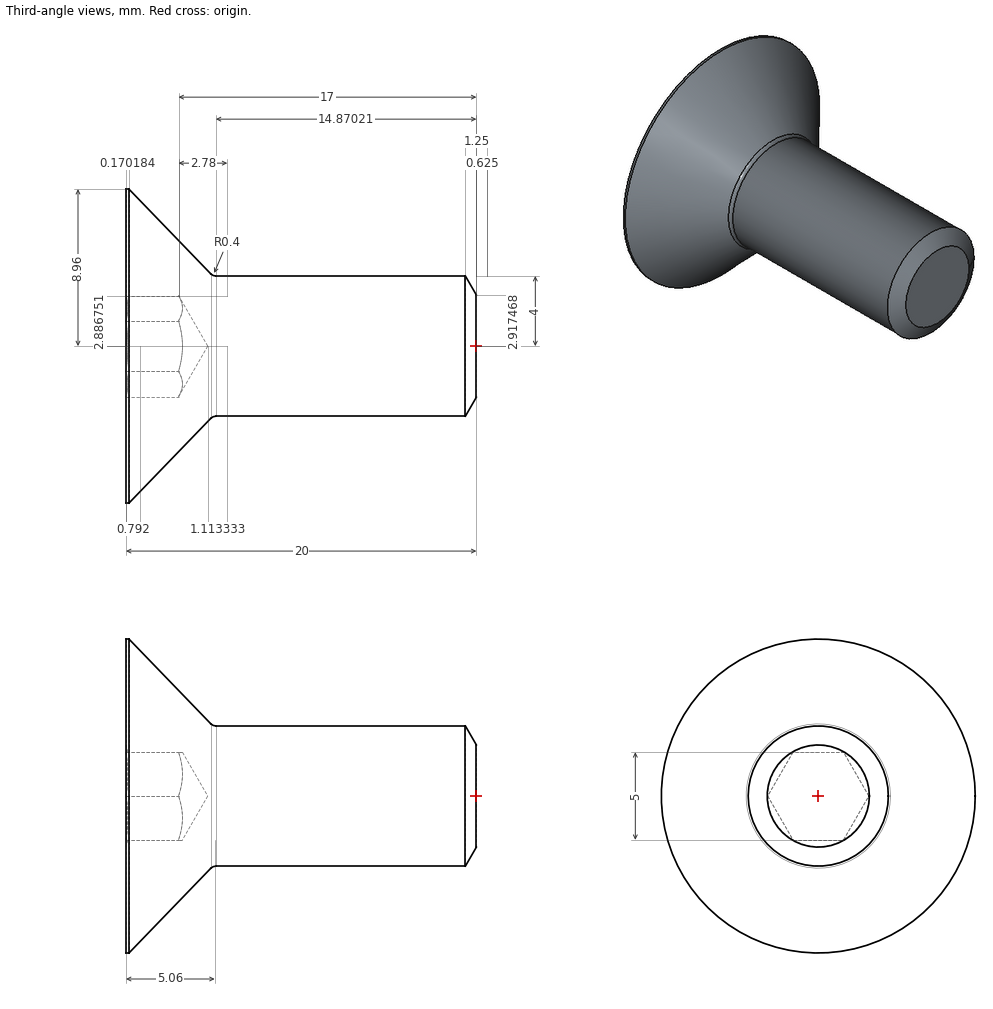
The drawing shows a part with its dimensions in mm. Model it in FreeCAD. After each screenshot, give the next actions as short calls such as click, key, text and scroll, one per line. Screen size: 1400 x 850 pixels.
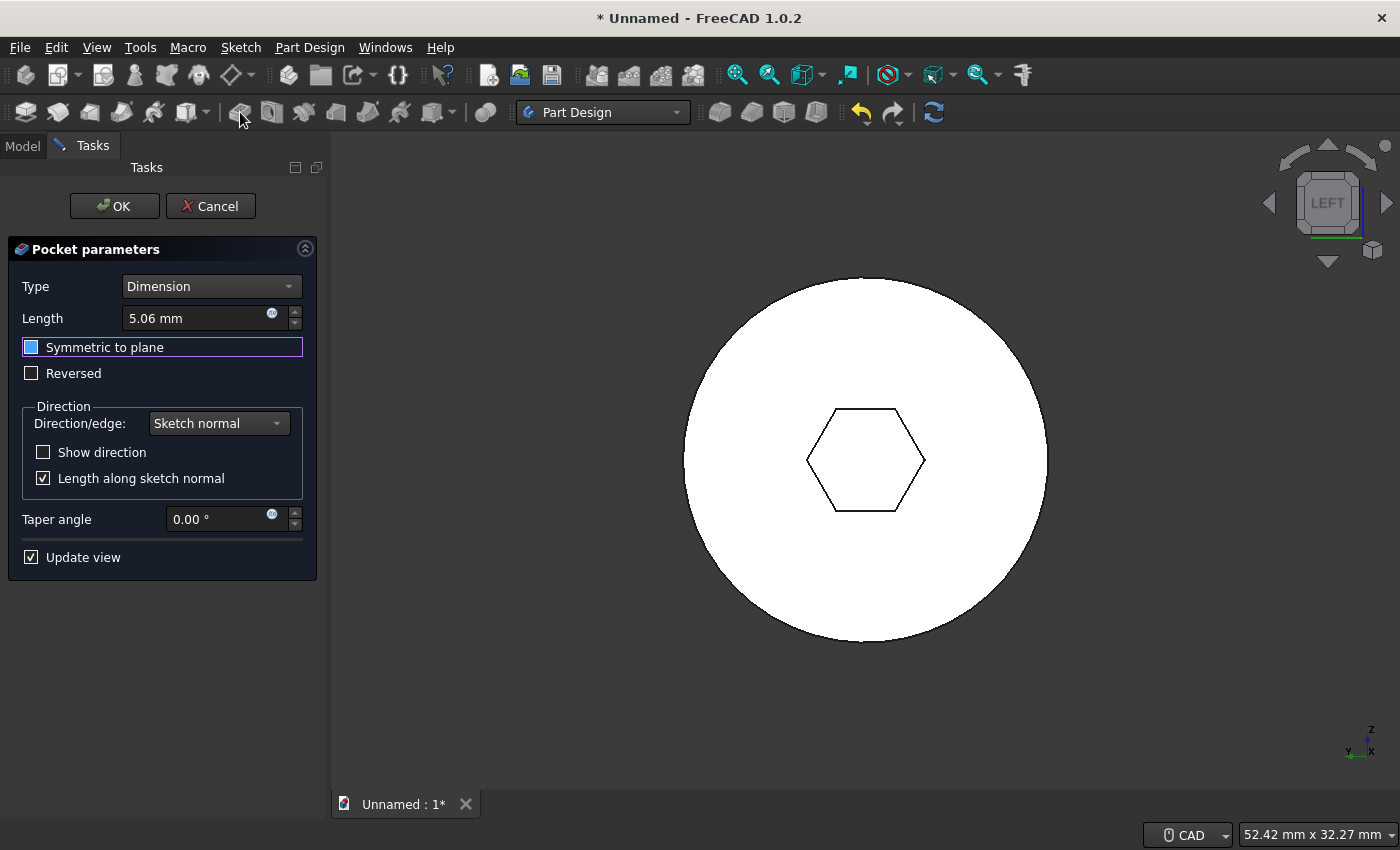
click(115, 206)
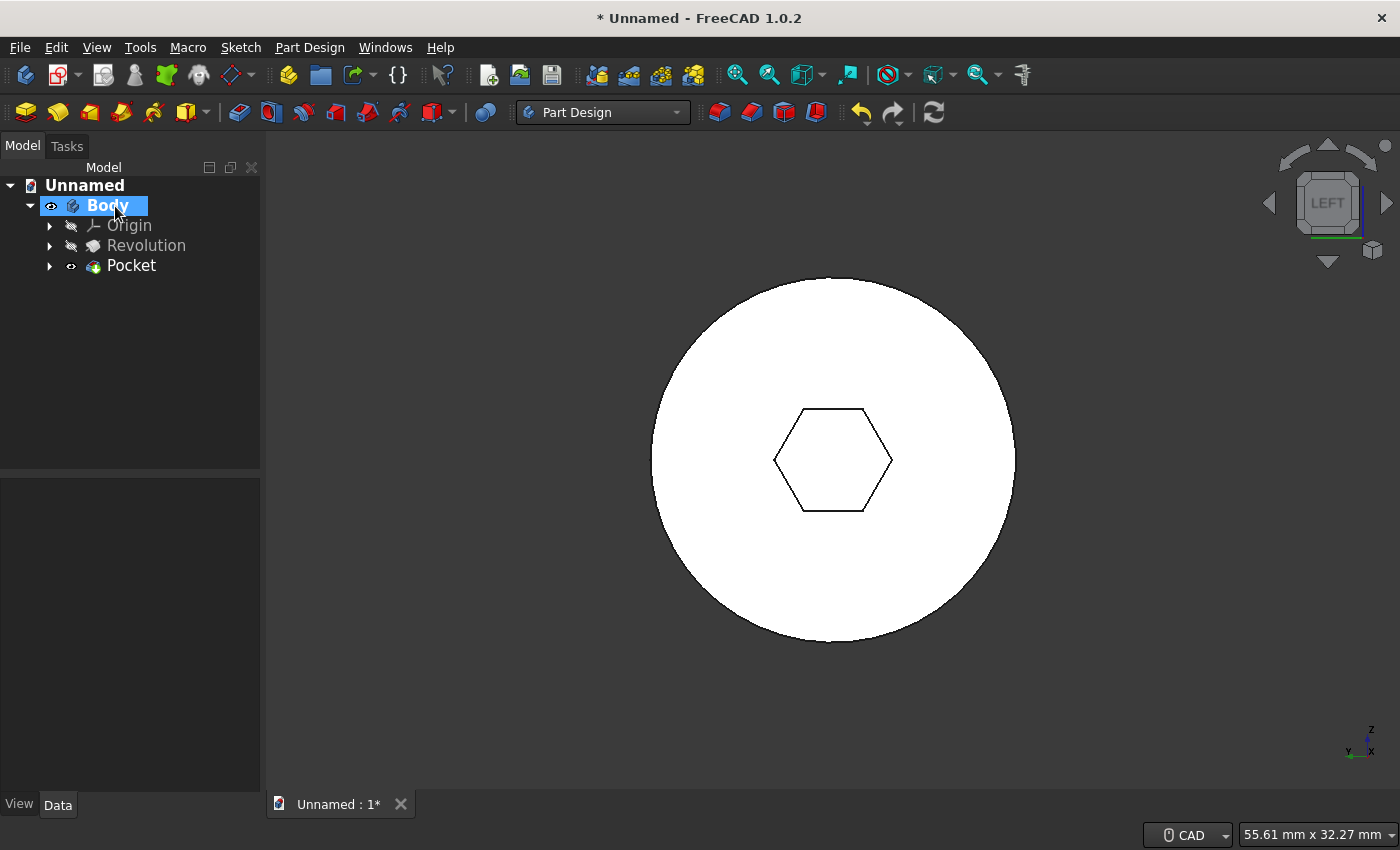
click(58, 76)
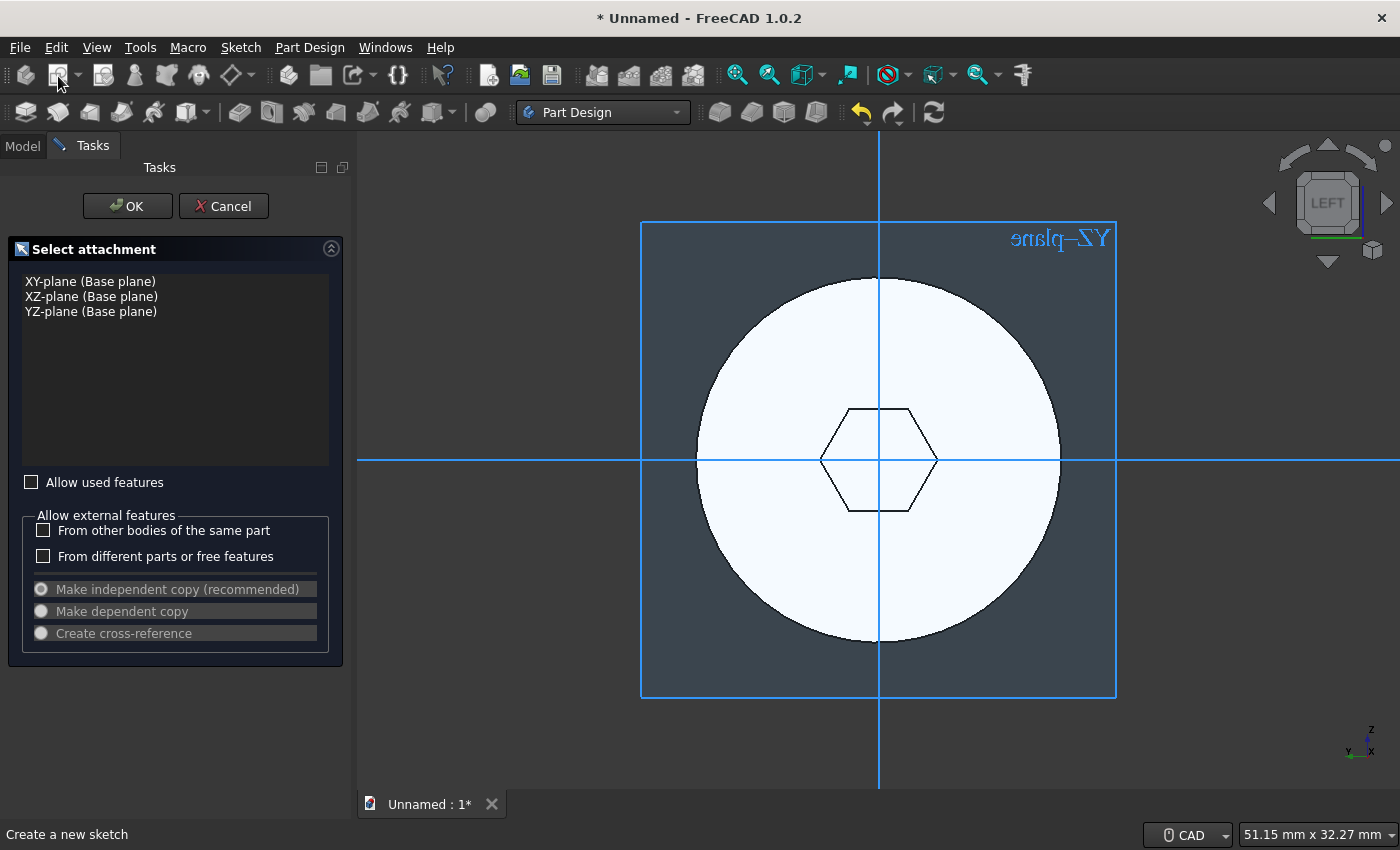
click(82, 282)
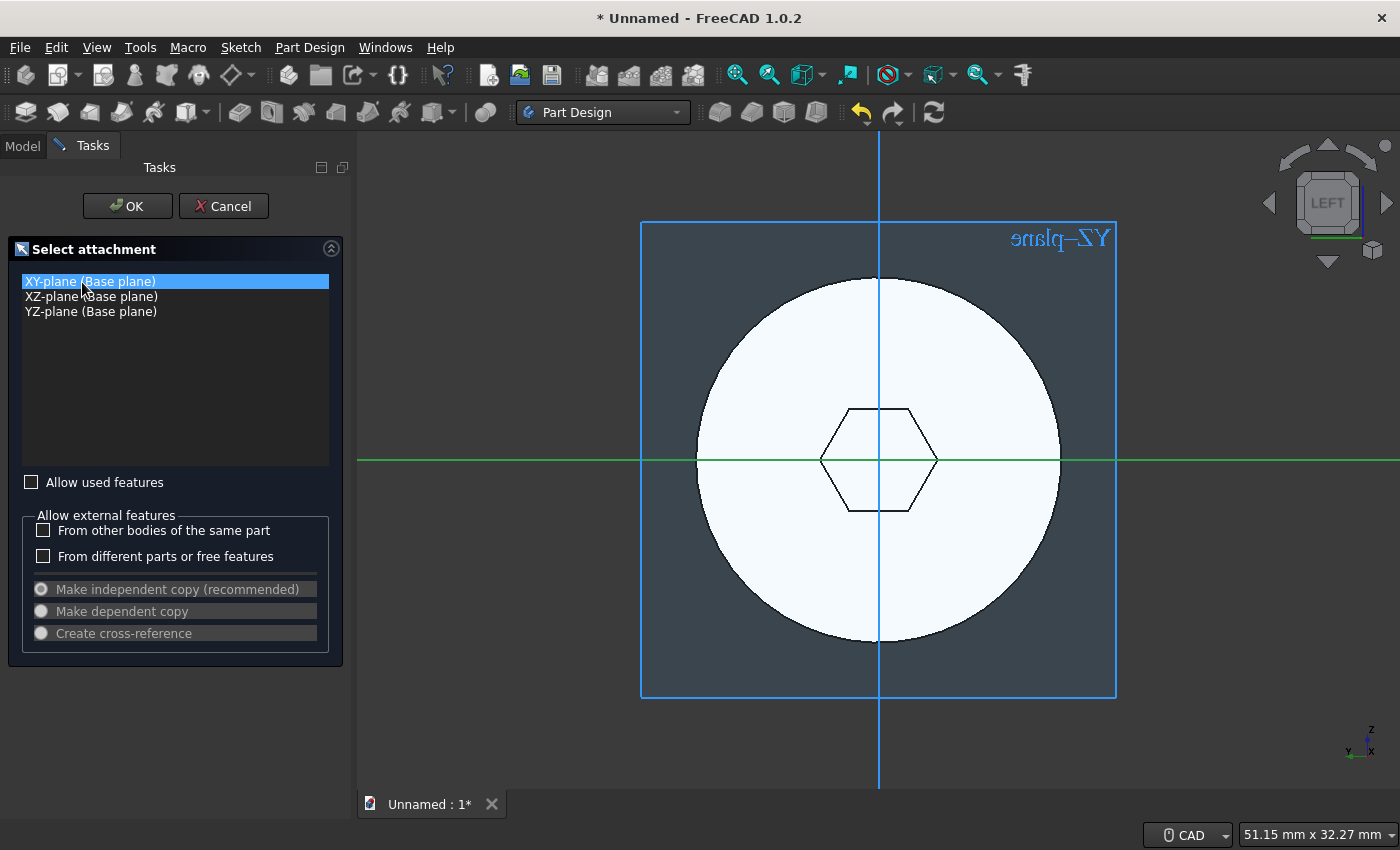
click(128, 206)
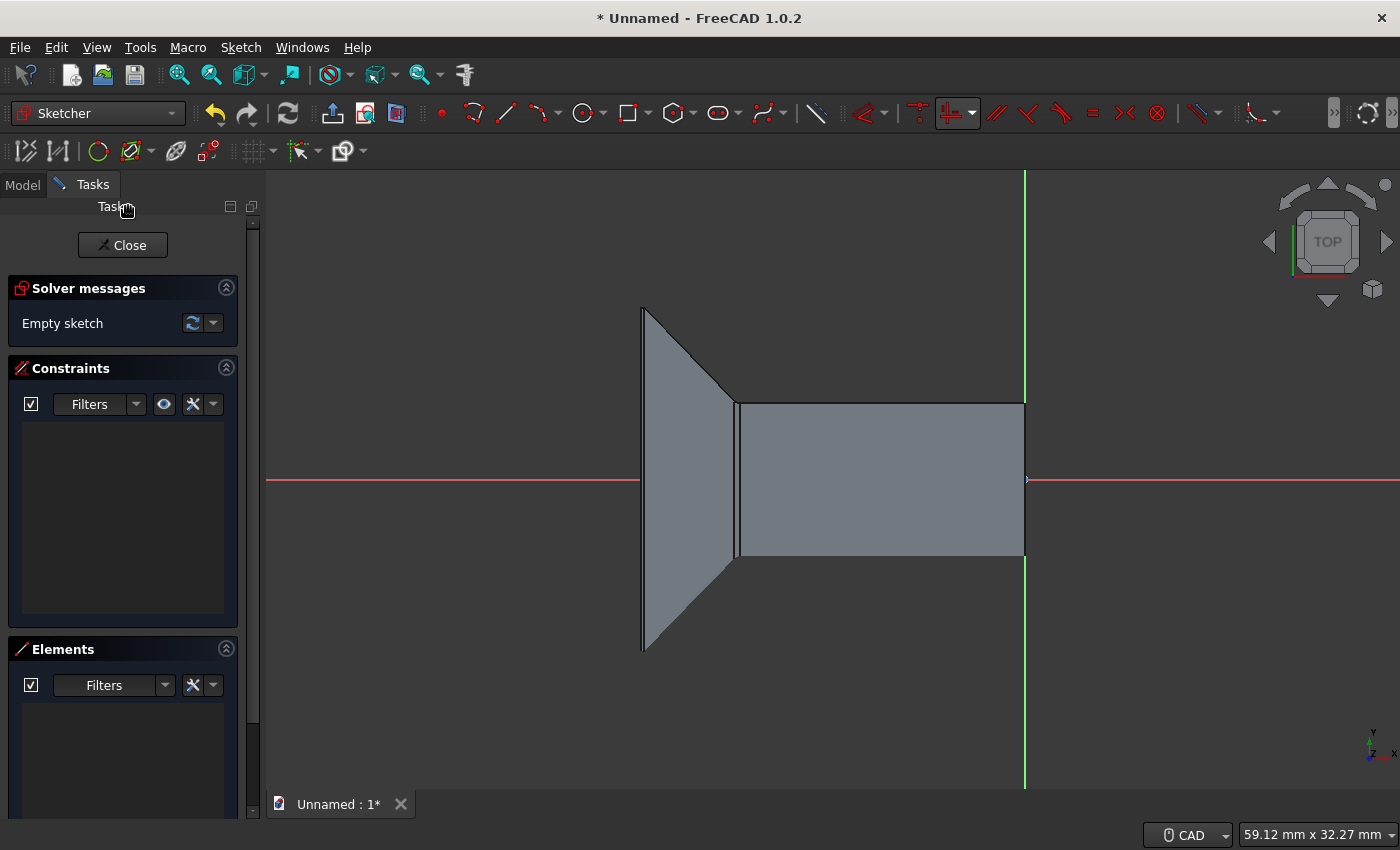
click(398, 114)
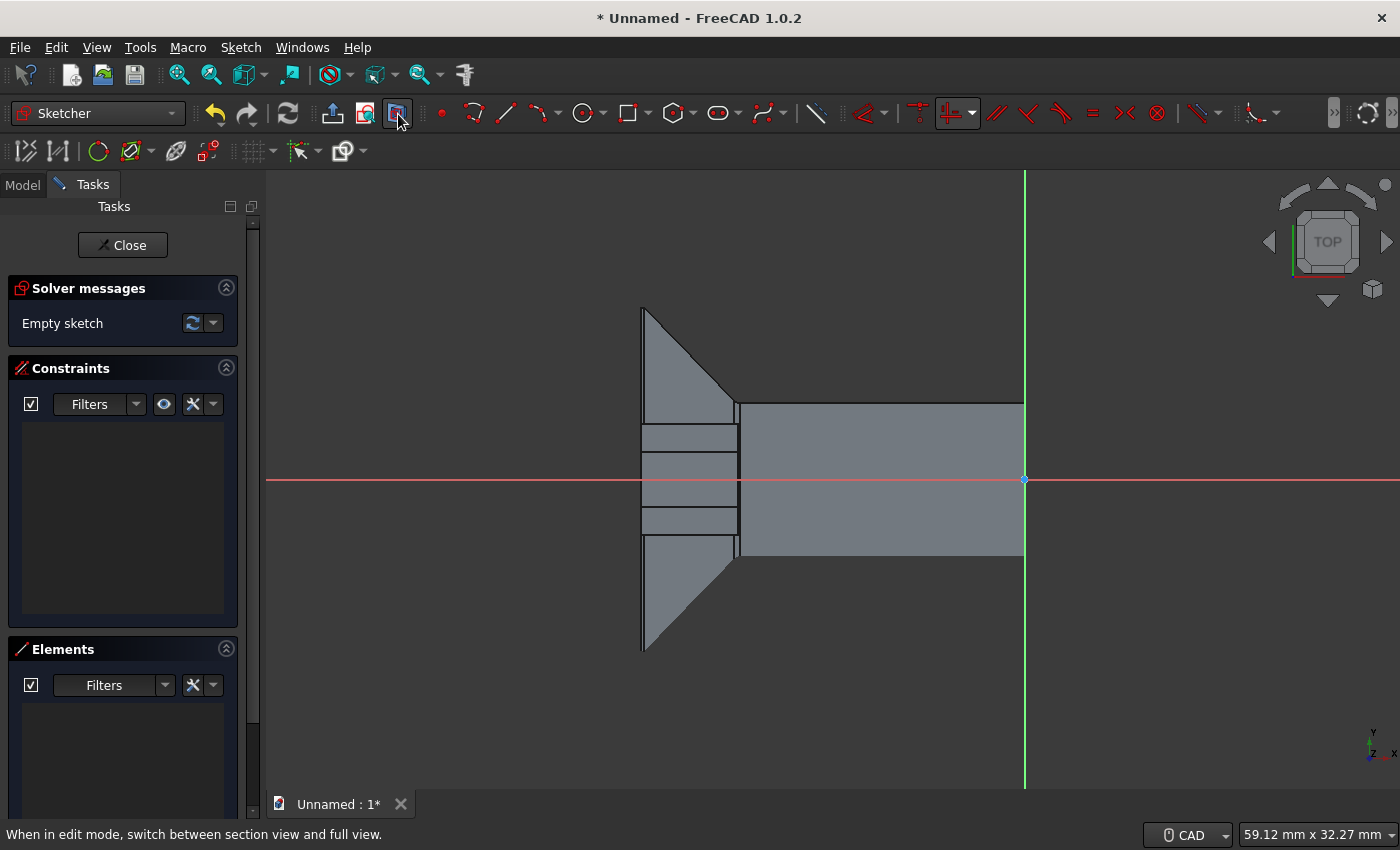
scroll(719, 448, up, 10)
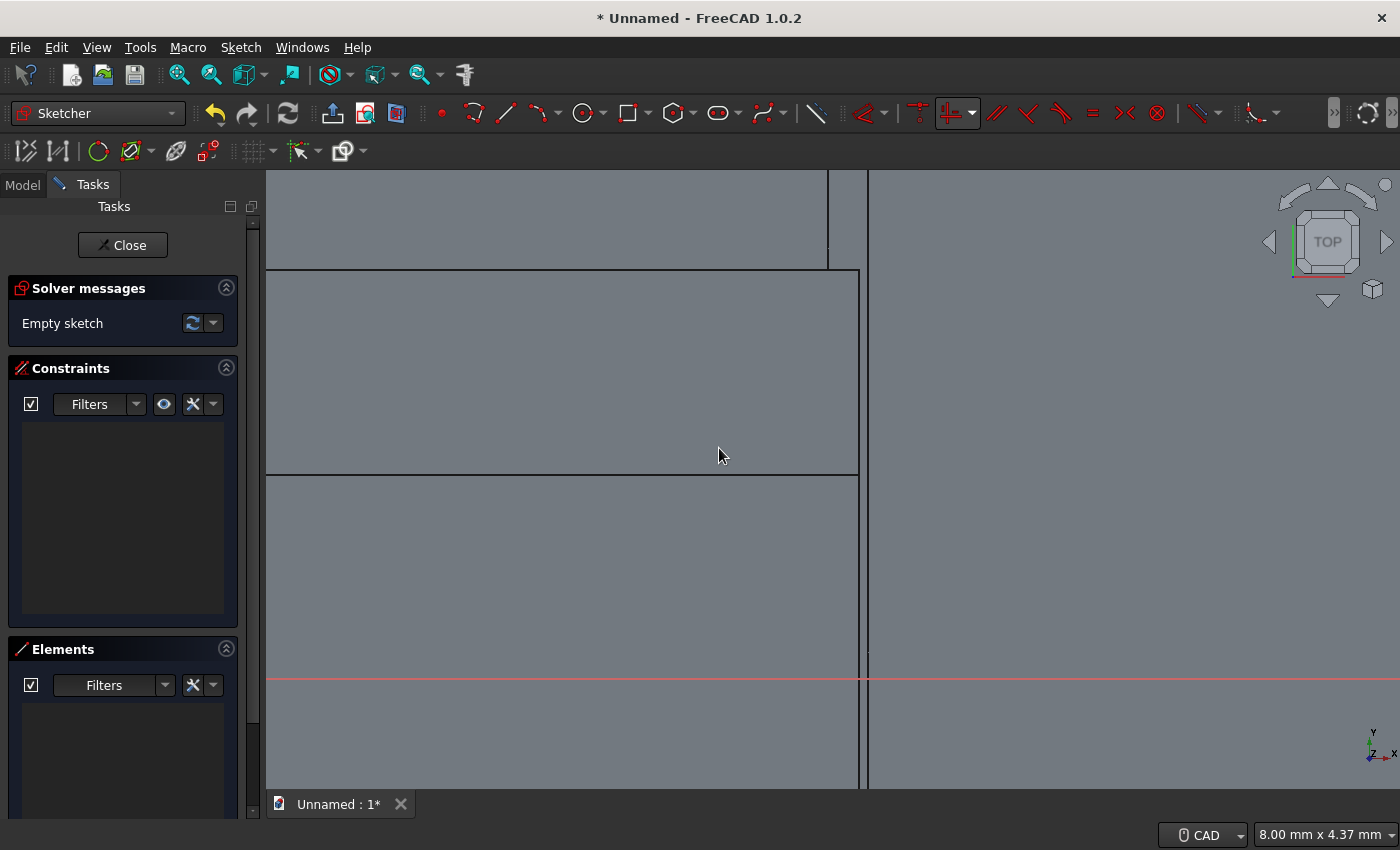
click(474, 114)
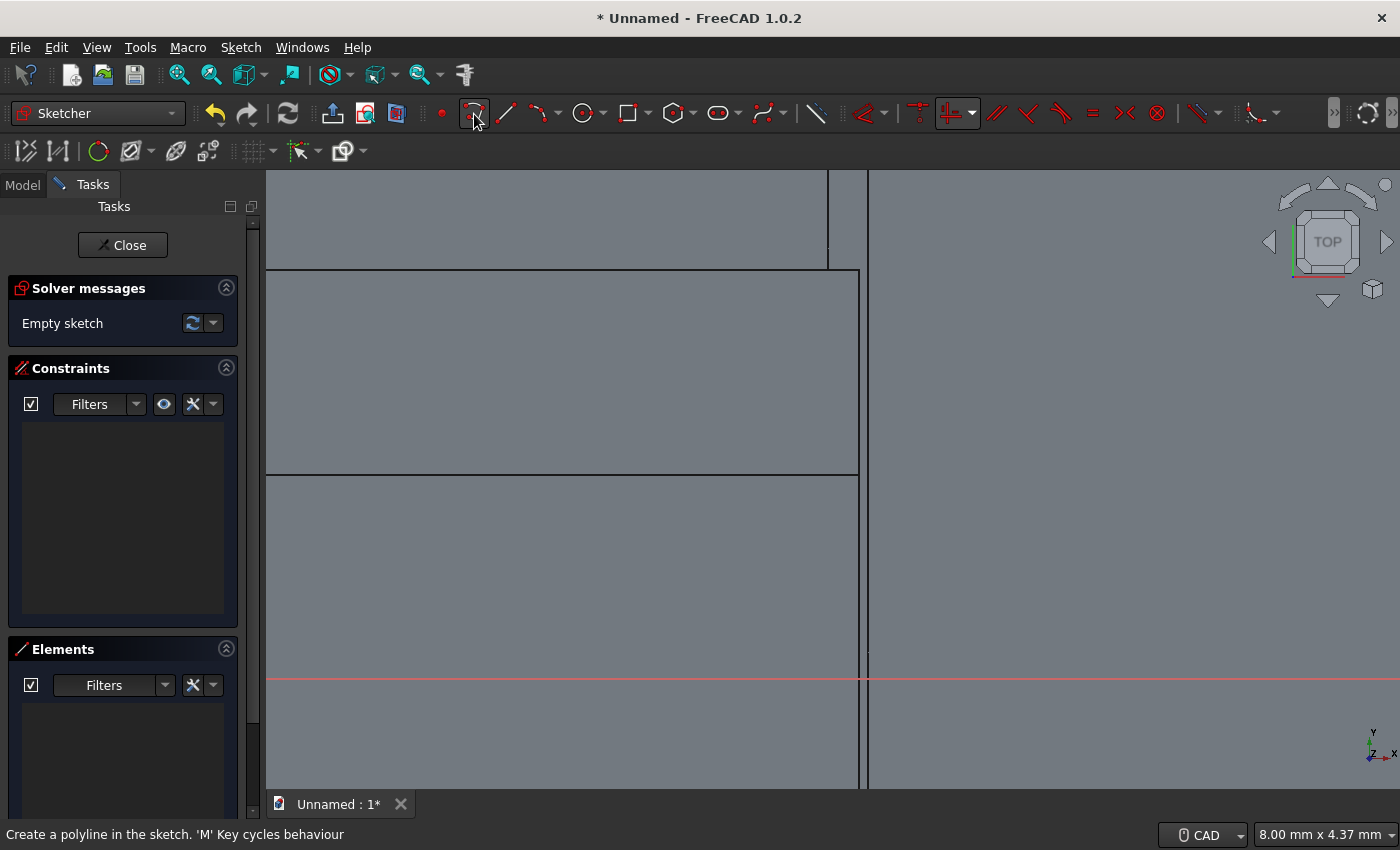
click(961, 679)
click(961, 270)
click(567, 270)
click(803, 670)
click(961, 679)
key(Escape)
key(Escape)